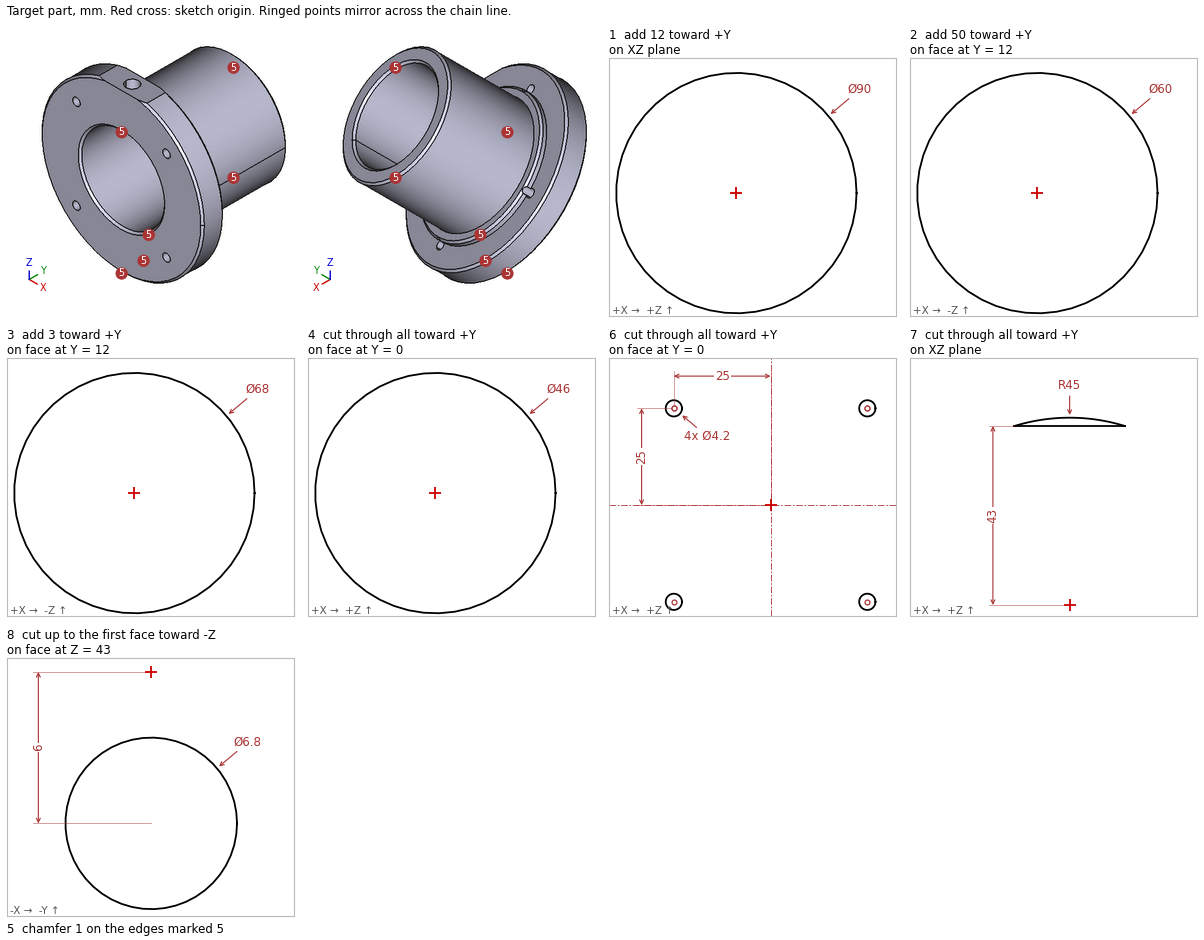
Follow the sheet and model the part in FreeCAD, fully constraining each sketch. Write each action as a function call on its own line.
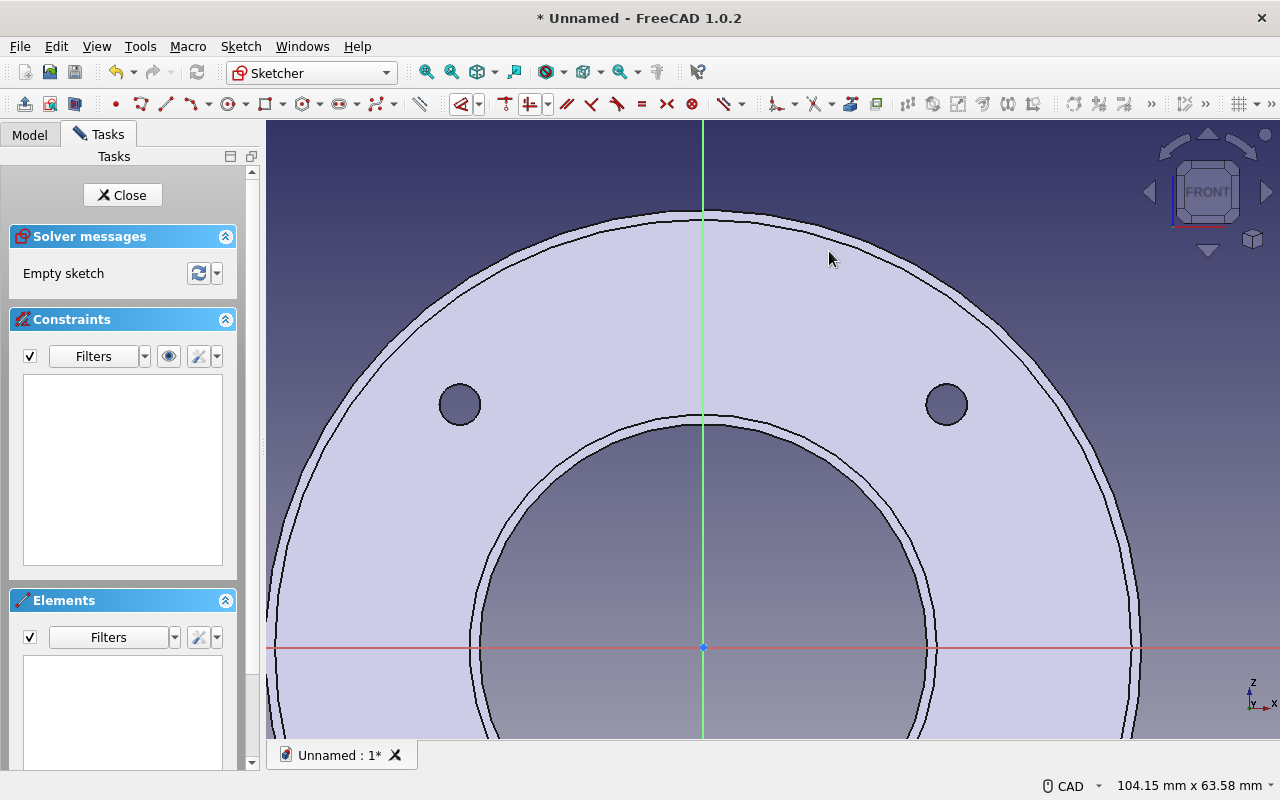
click(166, 104)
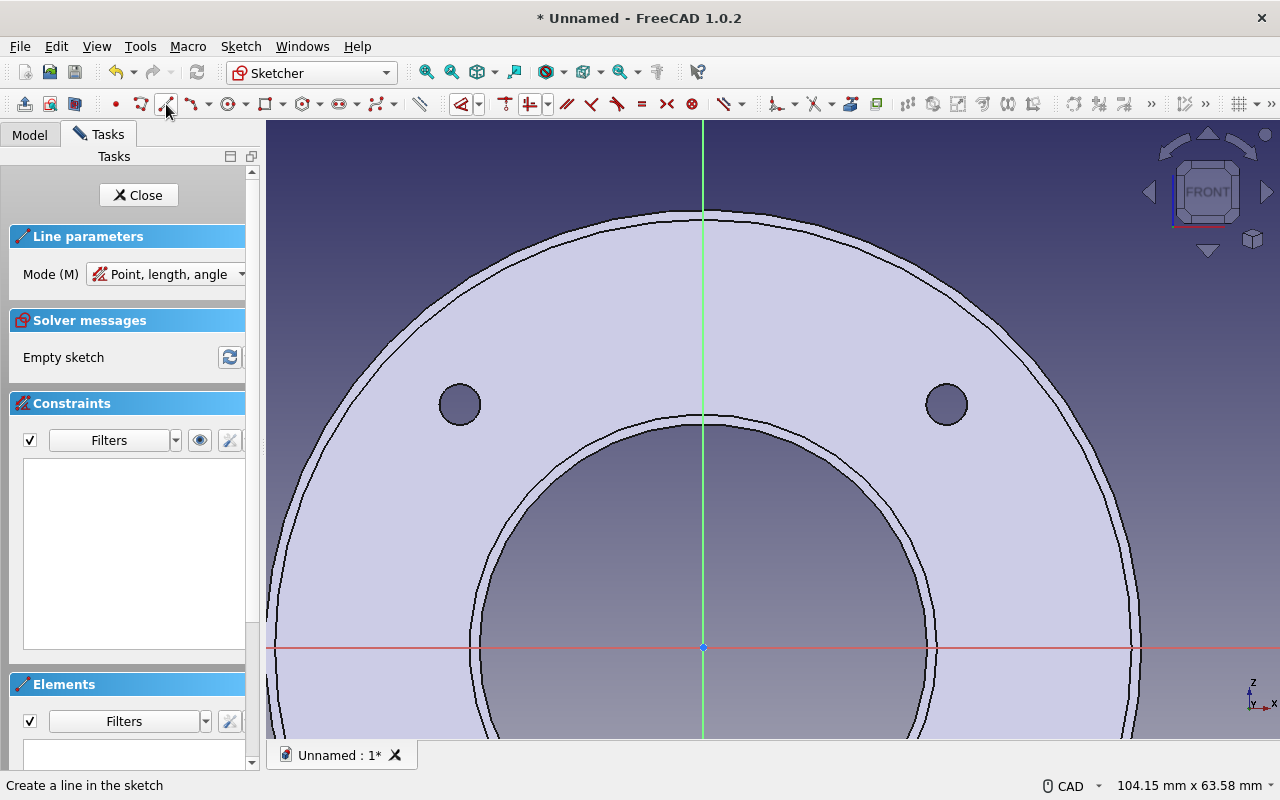
click(574, 229)
click(832, 229)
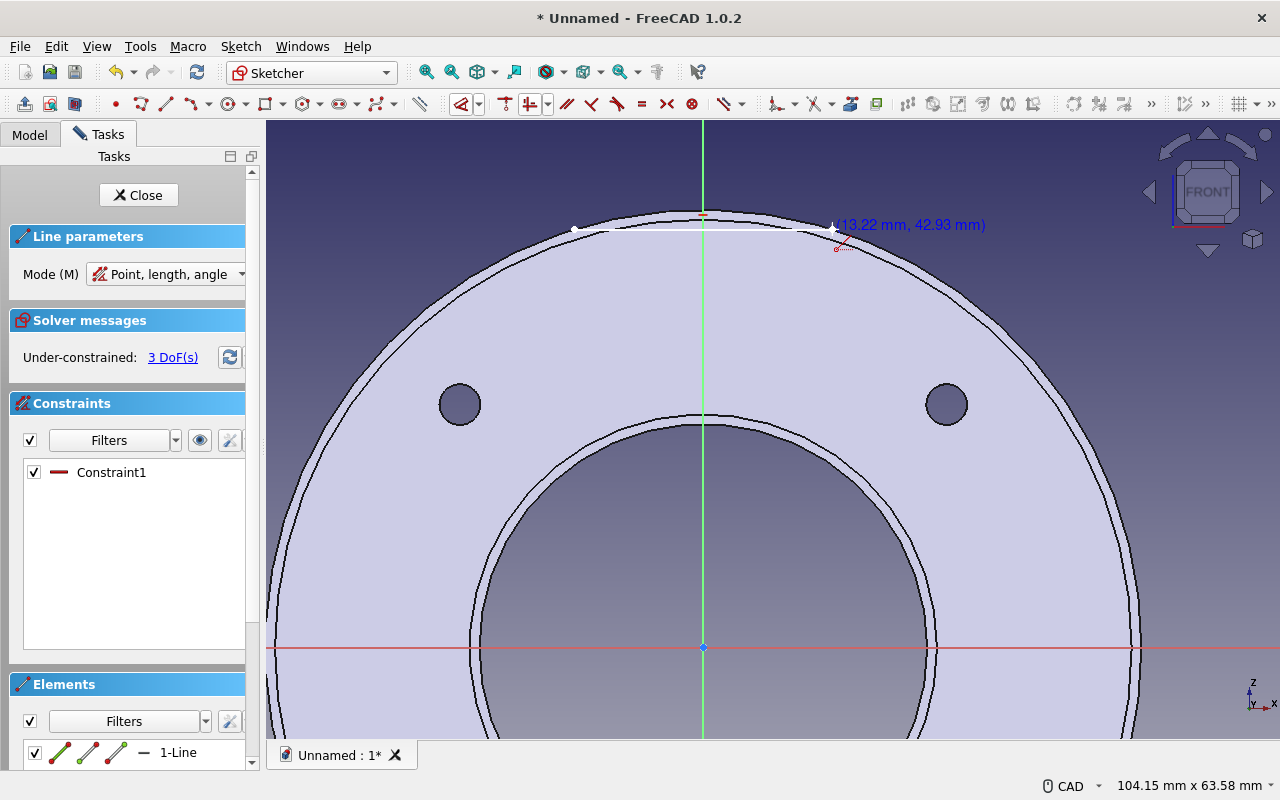
click(190, 104)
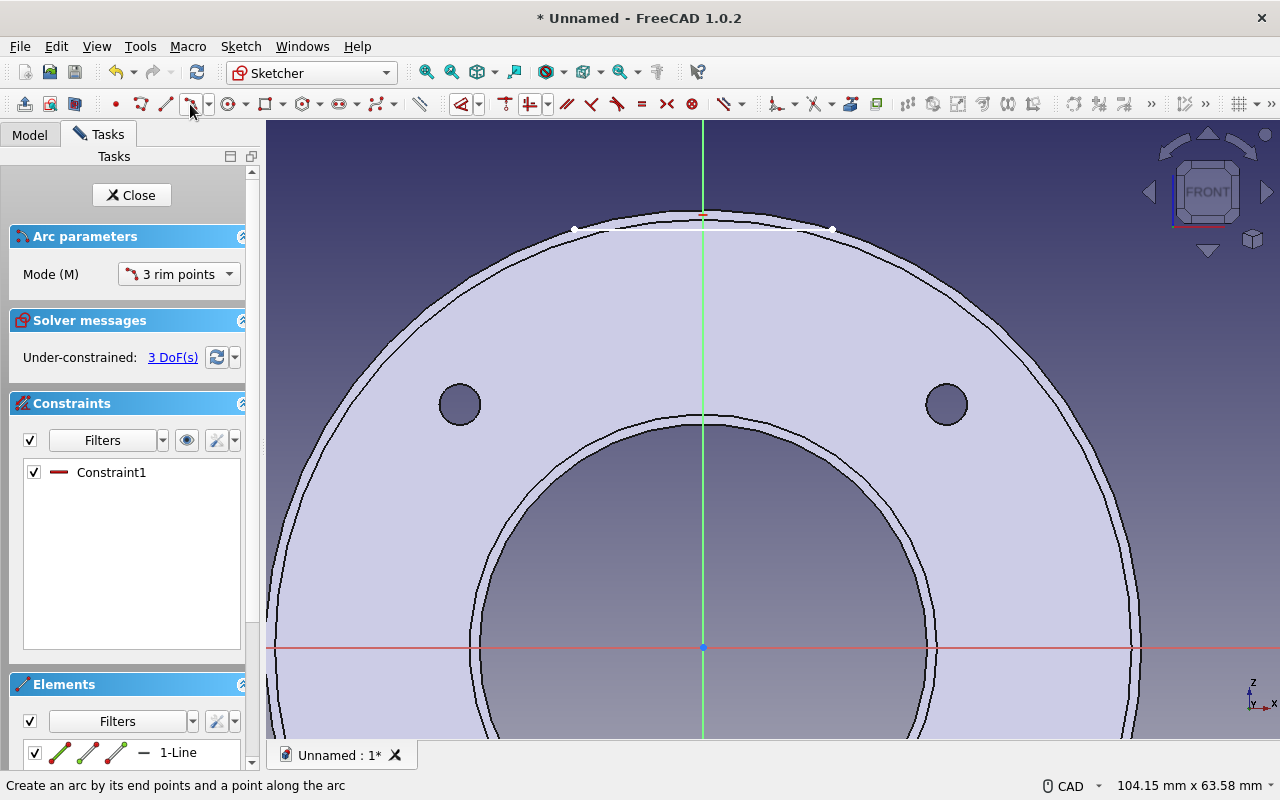
click(832, 230)
click(574, 230)
click(730, 211)
key(Escape)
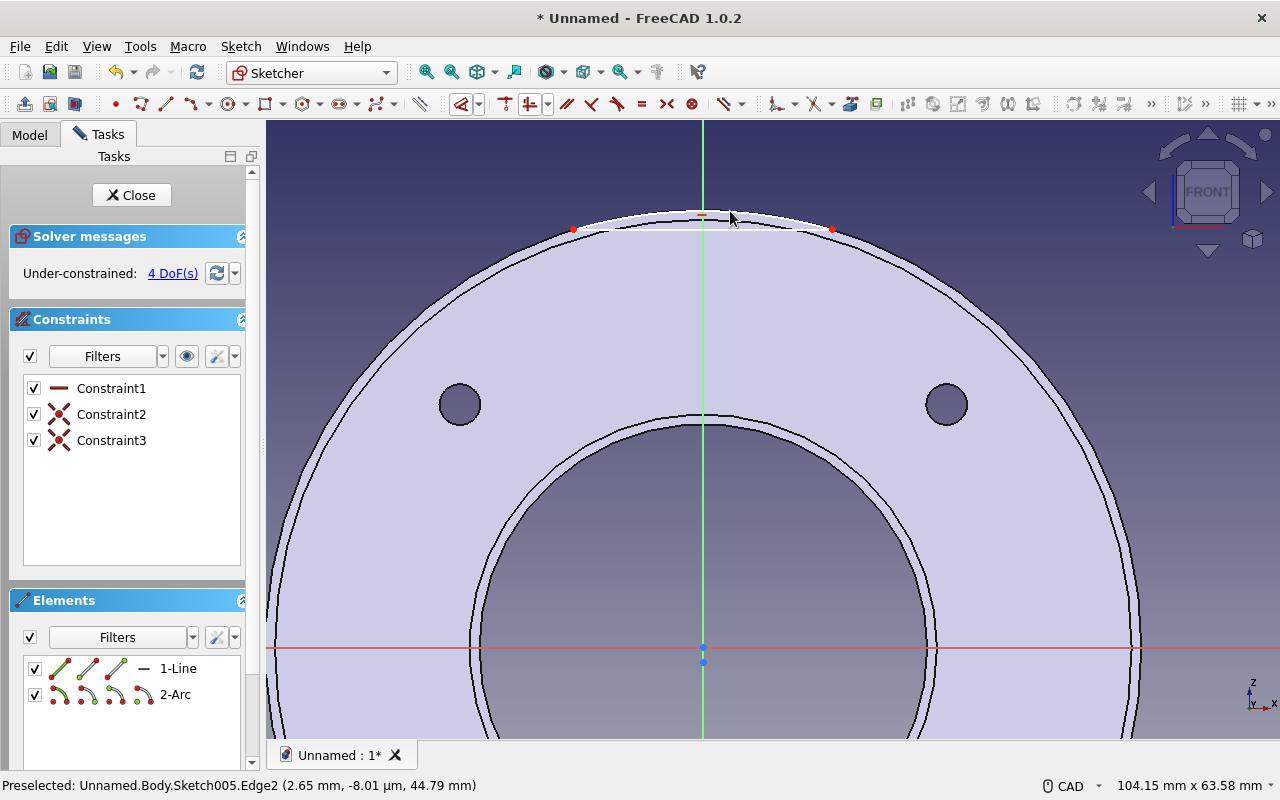
drag(693, 638, 713, 673)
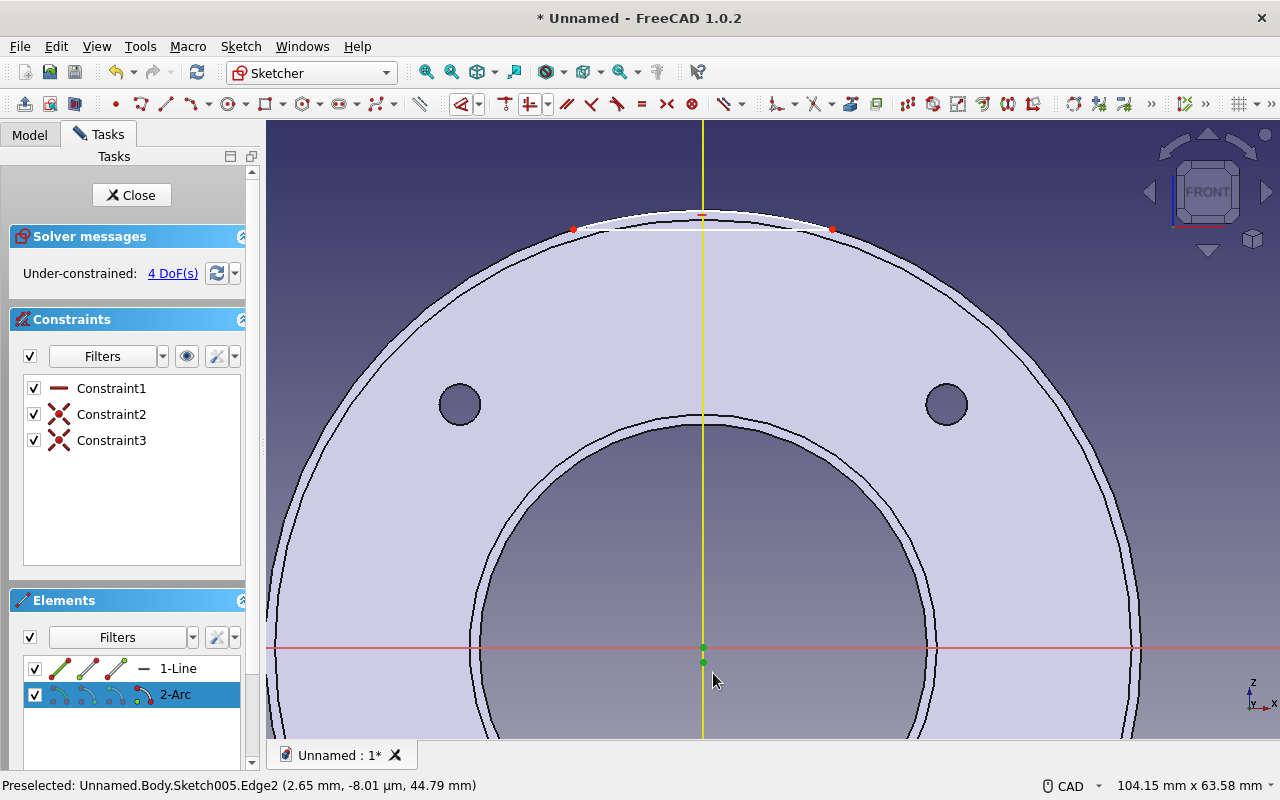
click(505, 104)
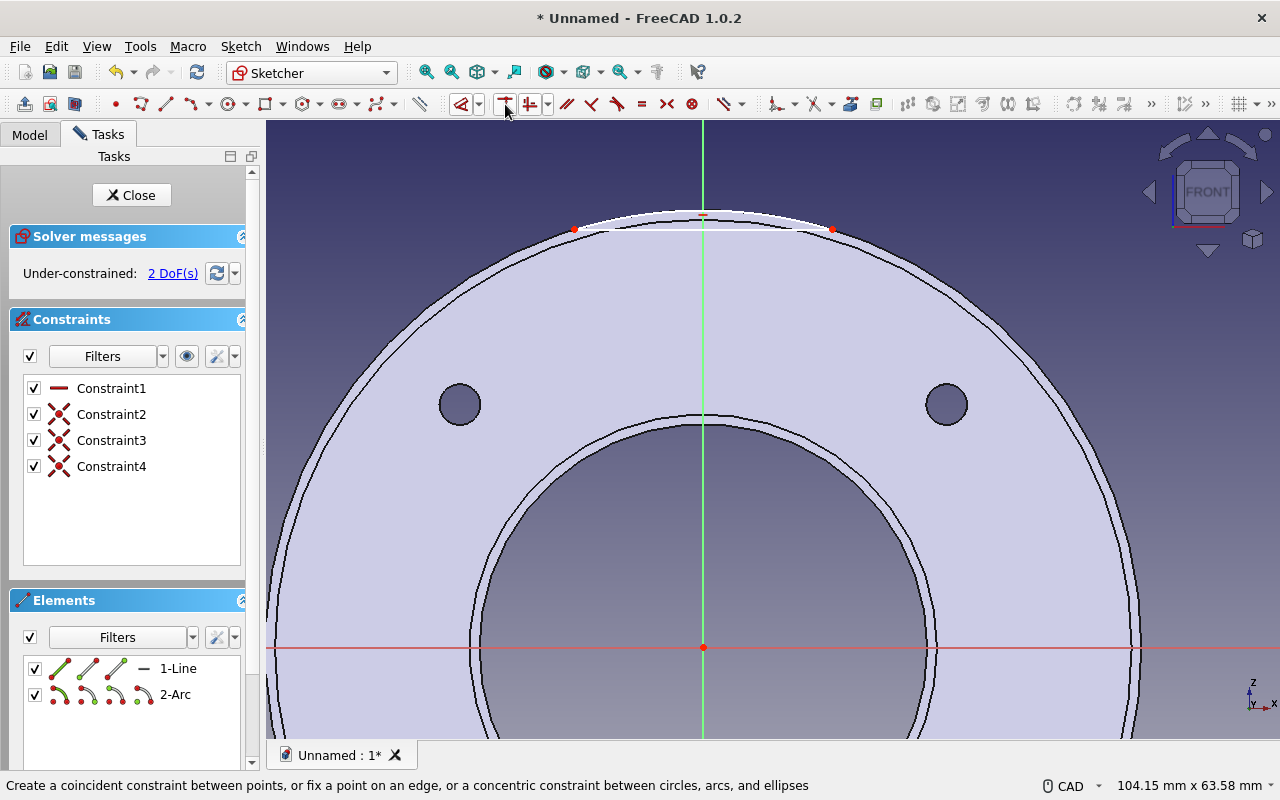
click(756, 214)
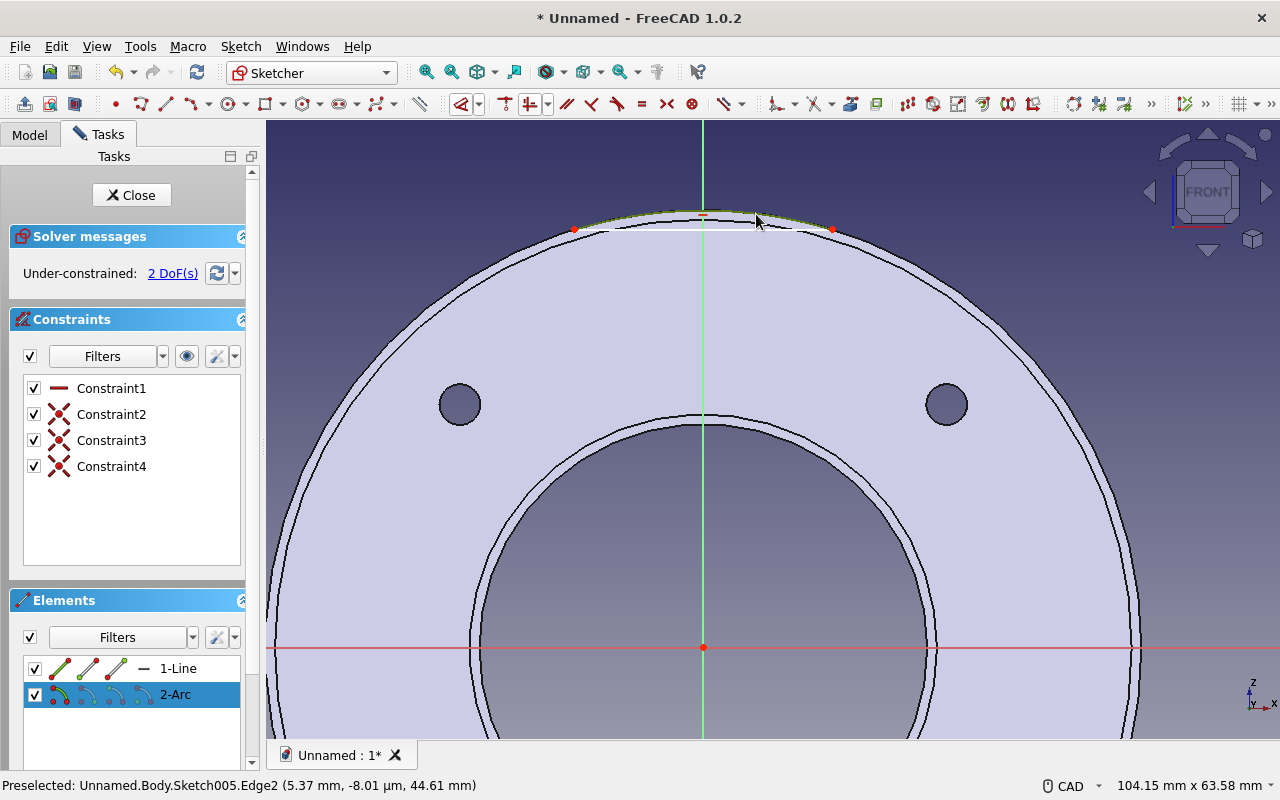
click(478, 104)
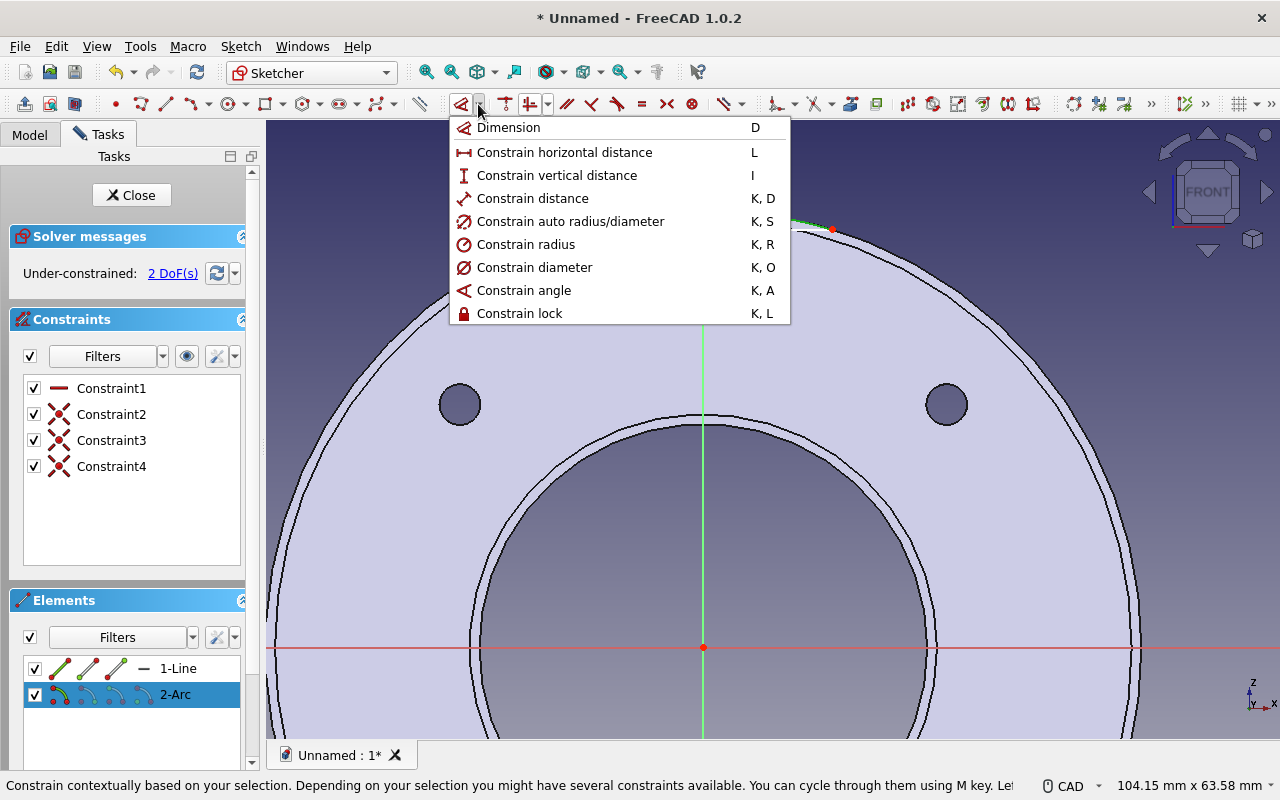
click(620, 244)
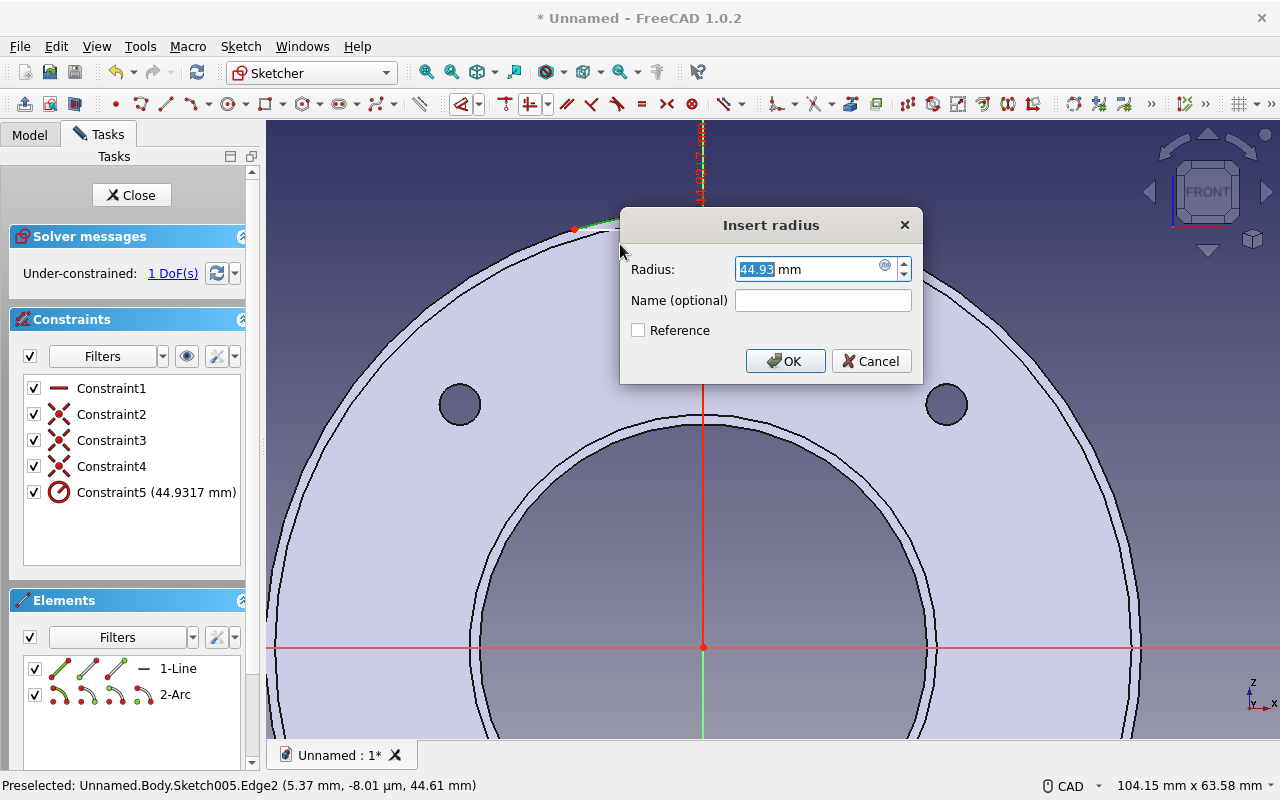
text(45)
key(Return)